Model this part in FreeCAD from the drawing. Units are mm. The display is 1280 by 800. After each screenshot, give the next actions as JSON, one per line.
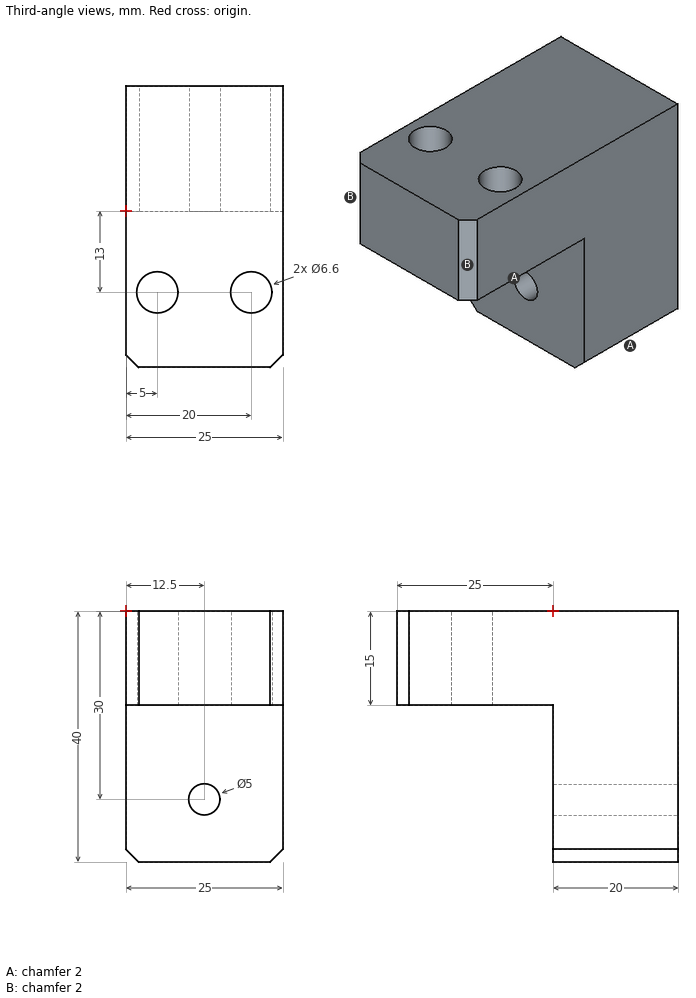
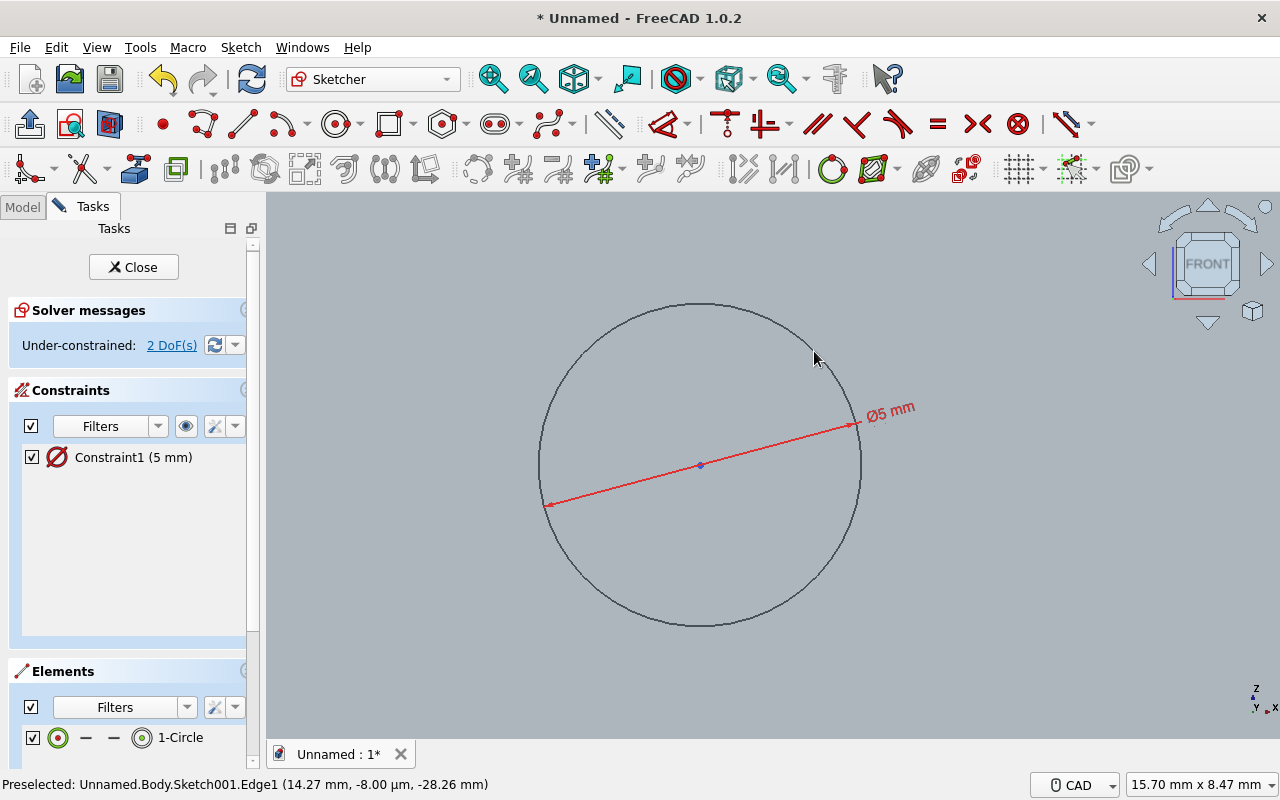
{"action": "left_click", "coordinate": [700, 465]}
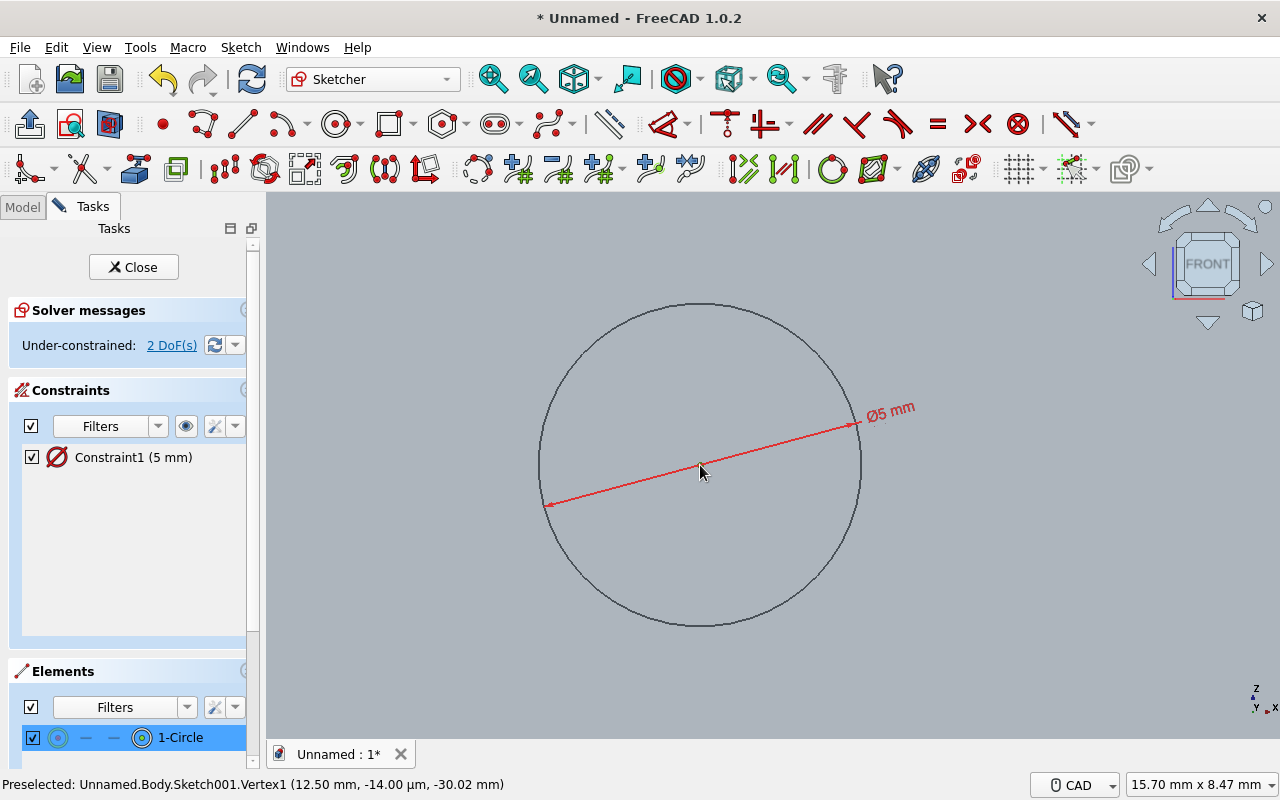
{"action": "key", "text": "i"}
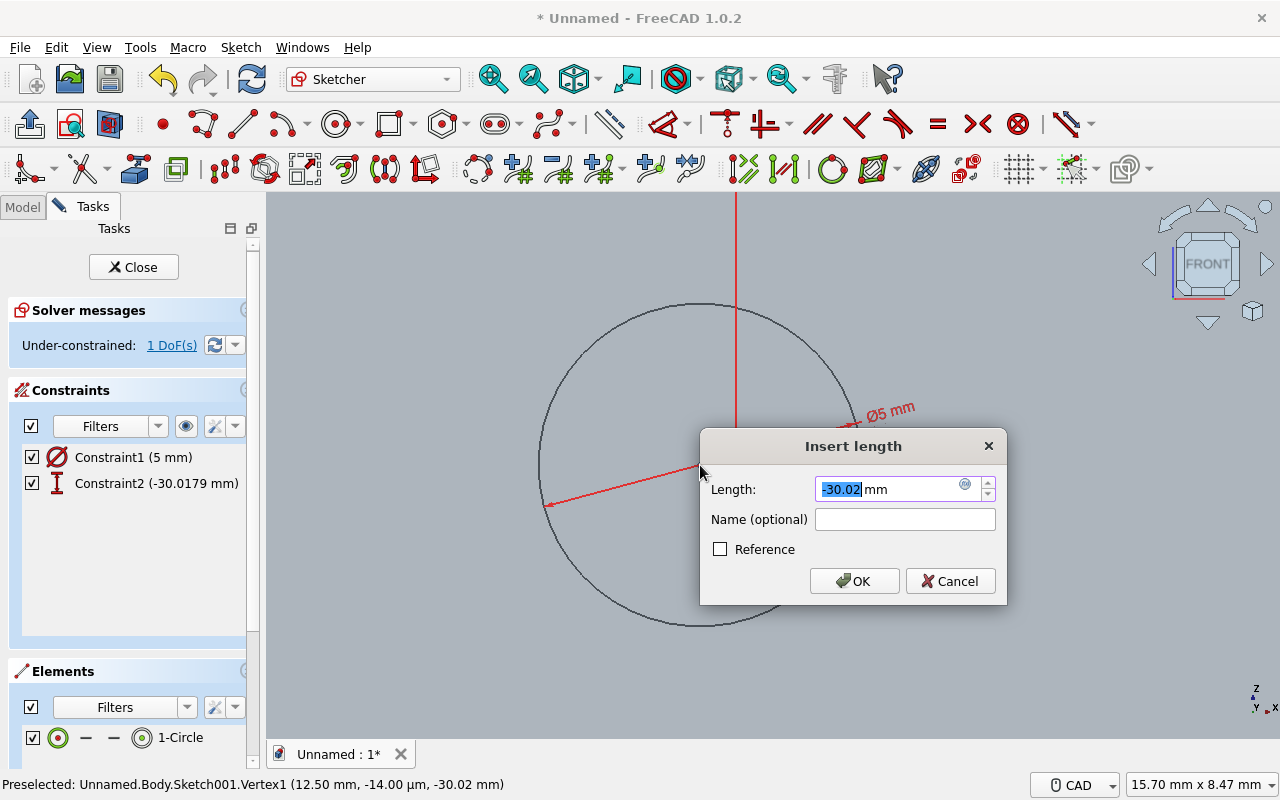
{"action": "type", "text": "-30"}
{"action": "key", "text": "Return"}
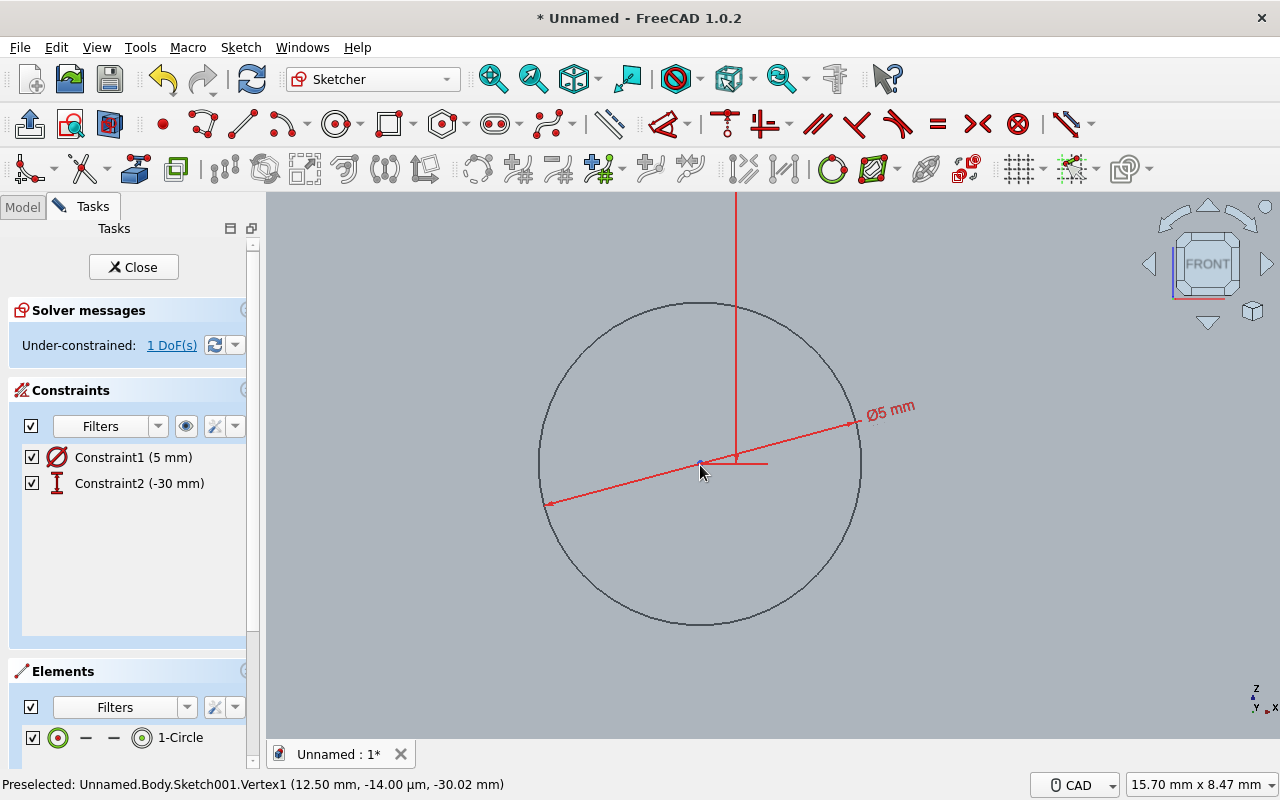
{"action": "left_click", "coordinate": [700, 464]}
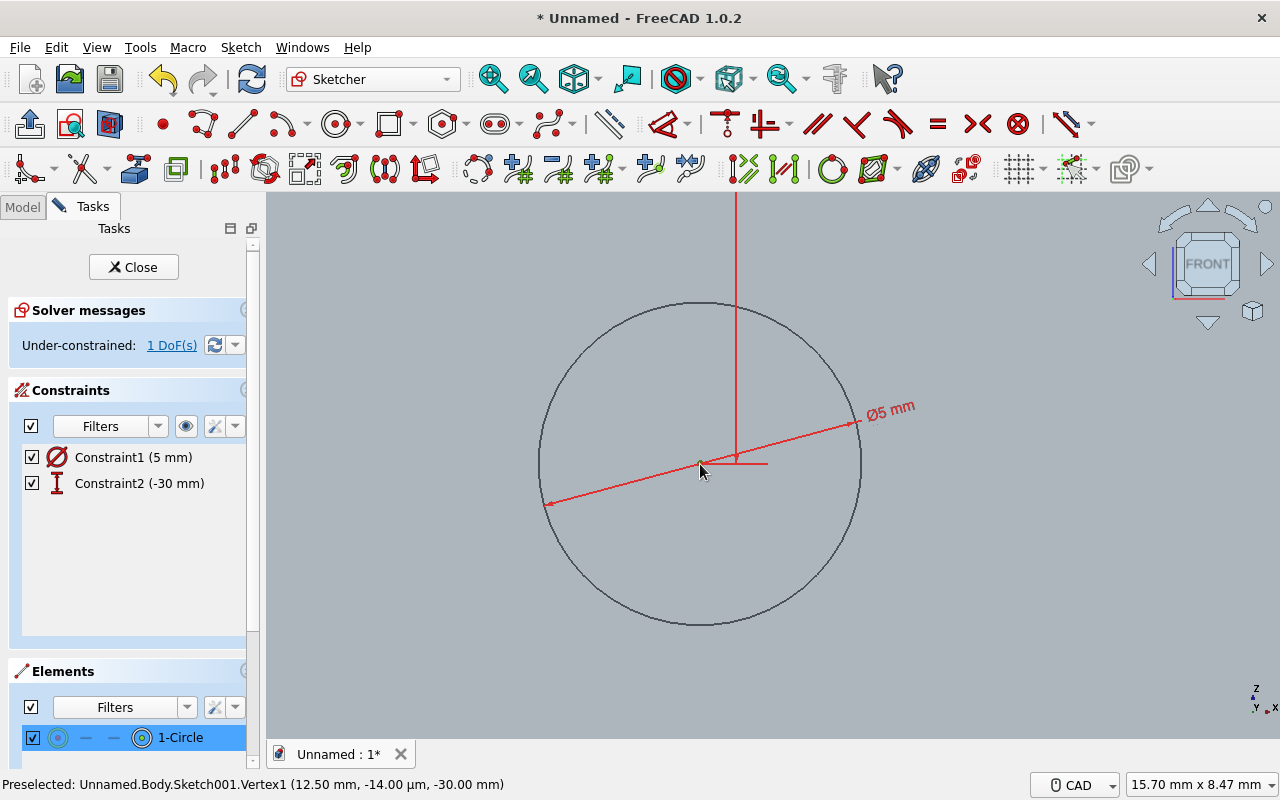
{"action": "key", "text": "l"}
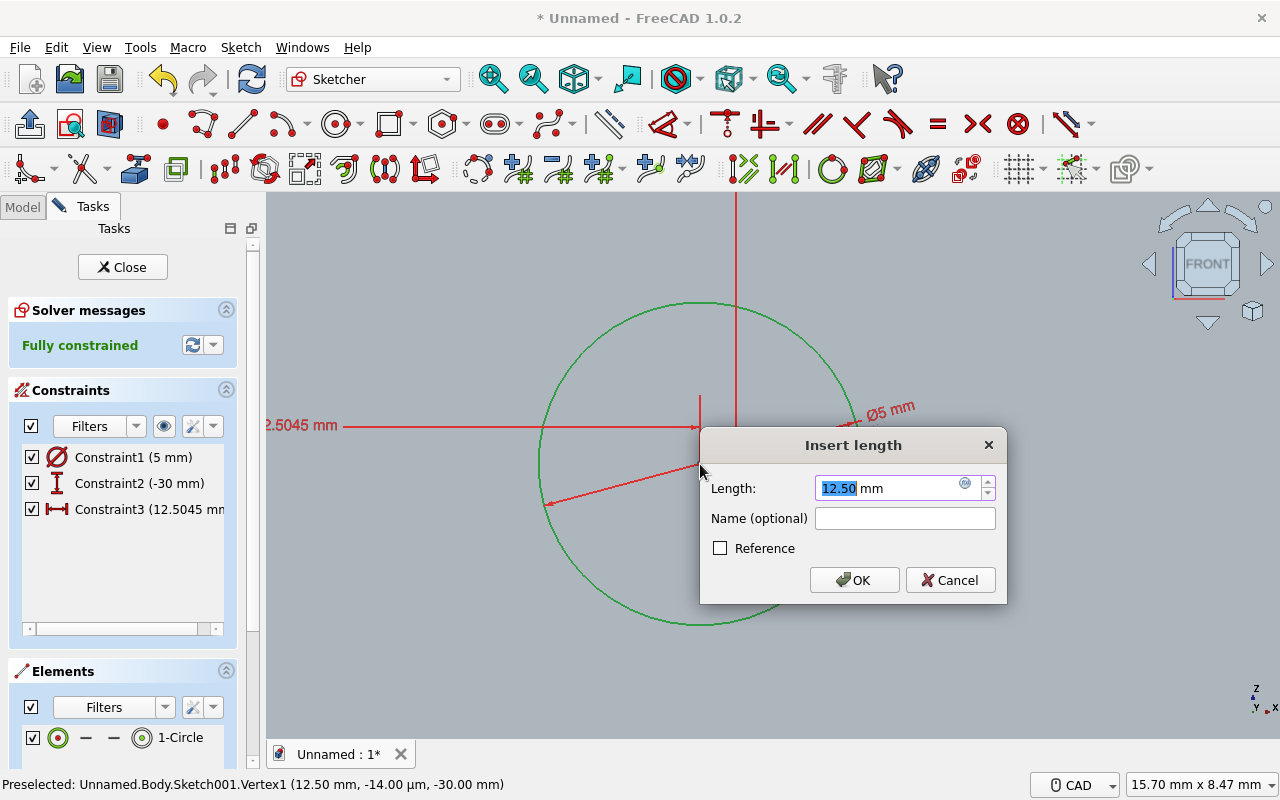
{"action": "type", "text": "12.5"}
{"action": "key", "text": "Return"}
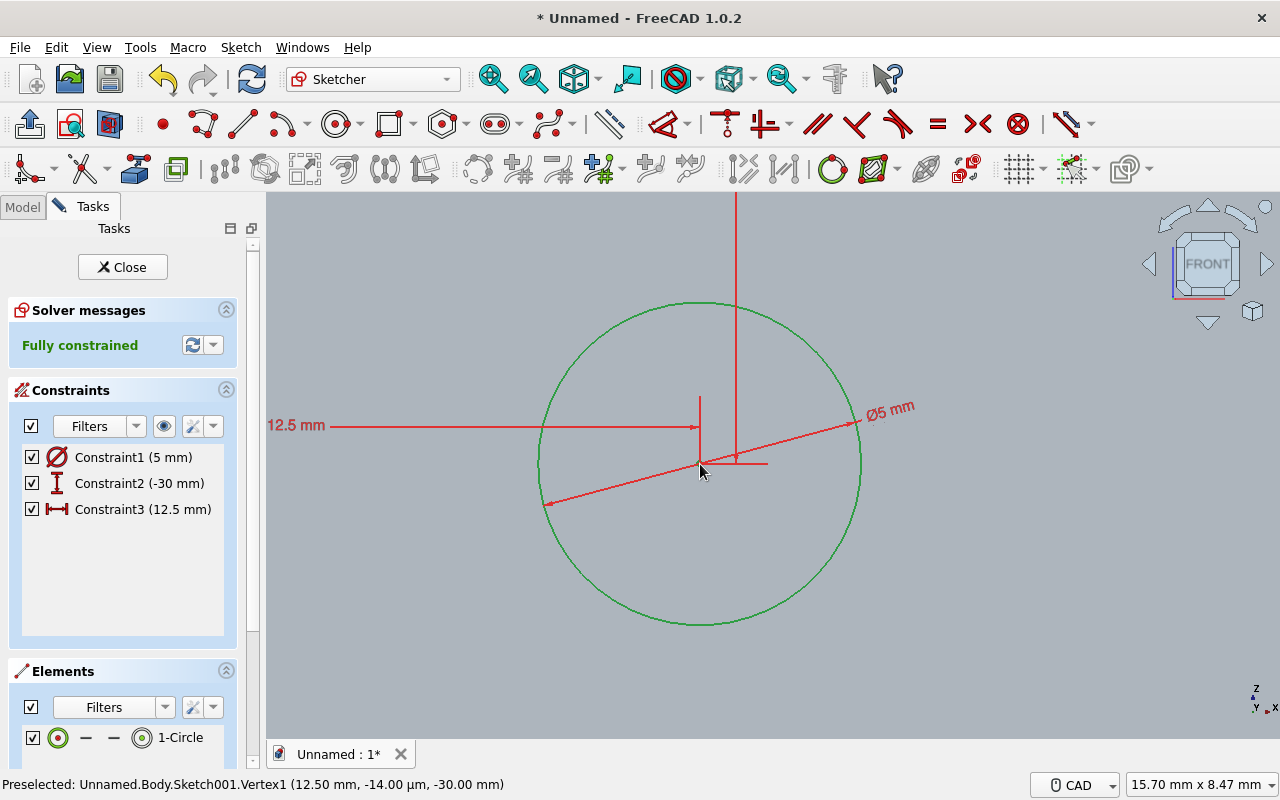
{"action": "left_click", "coordinate": [123, 267]}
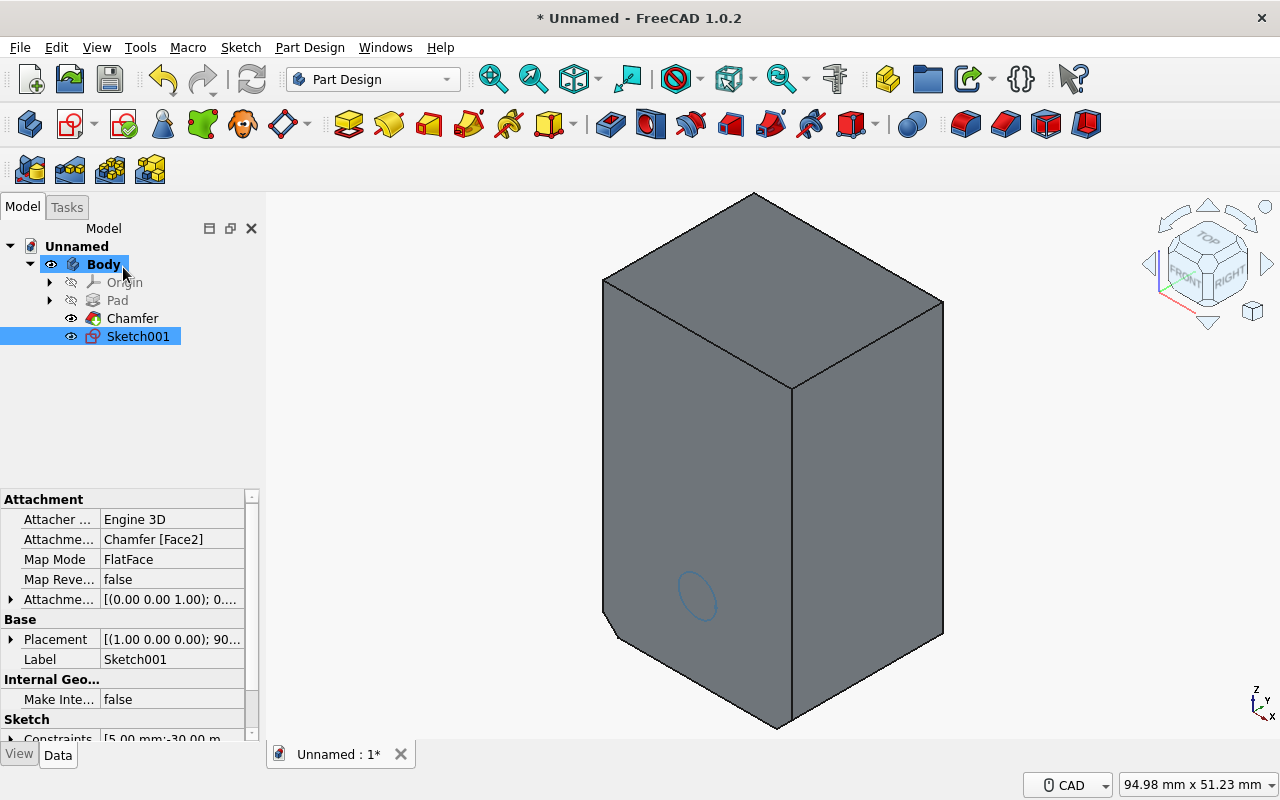
{"action": "left_click", "coordinate": [612, 124]}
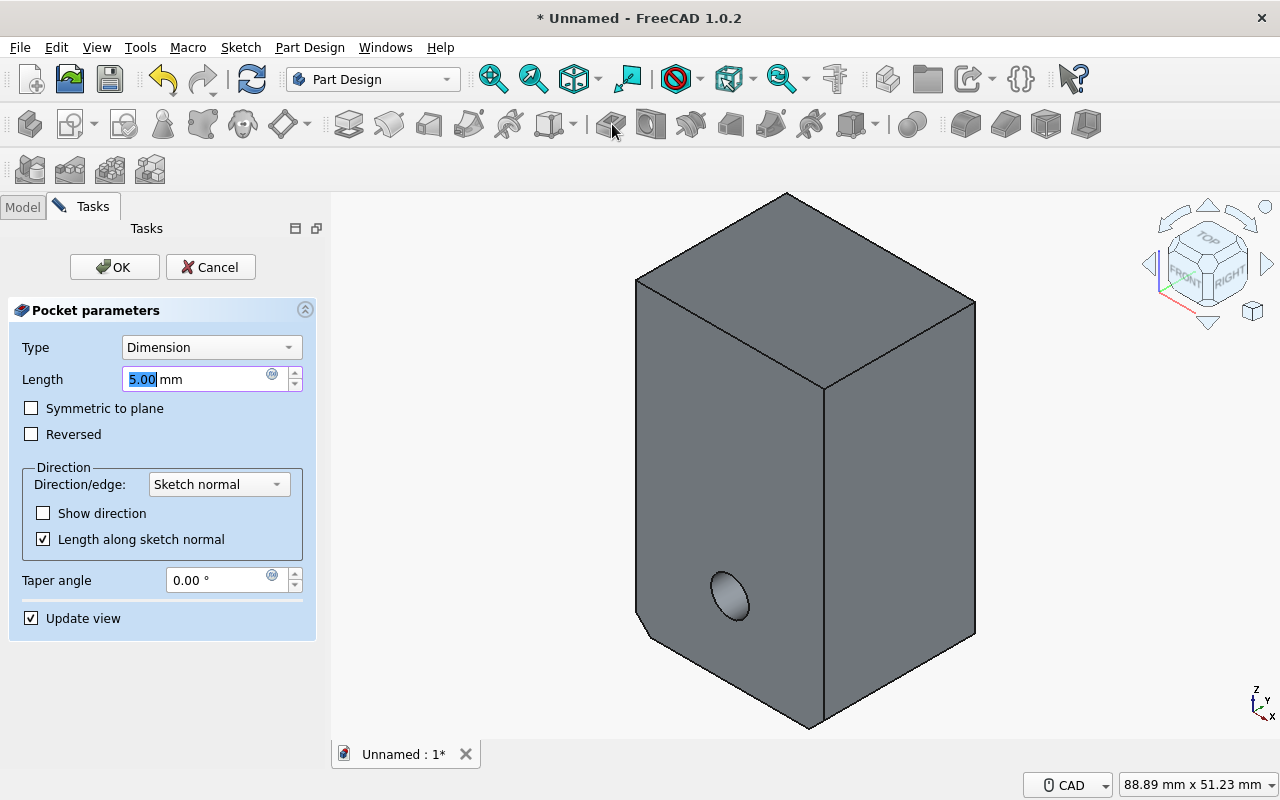
{"action": "left_click", "coordinate": [212, 348]}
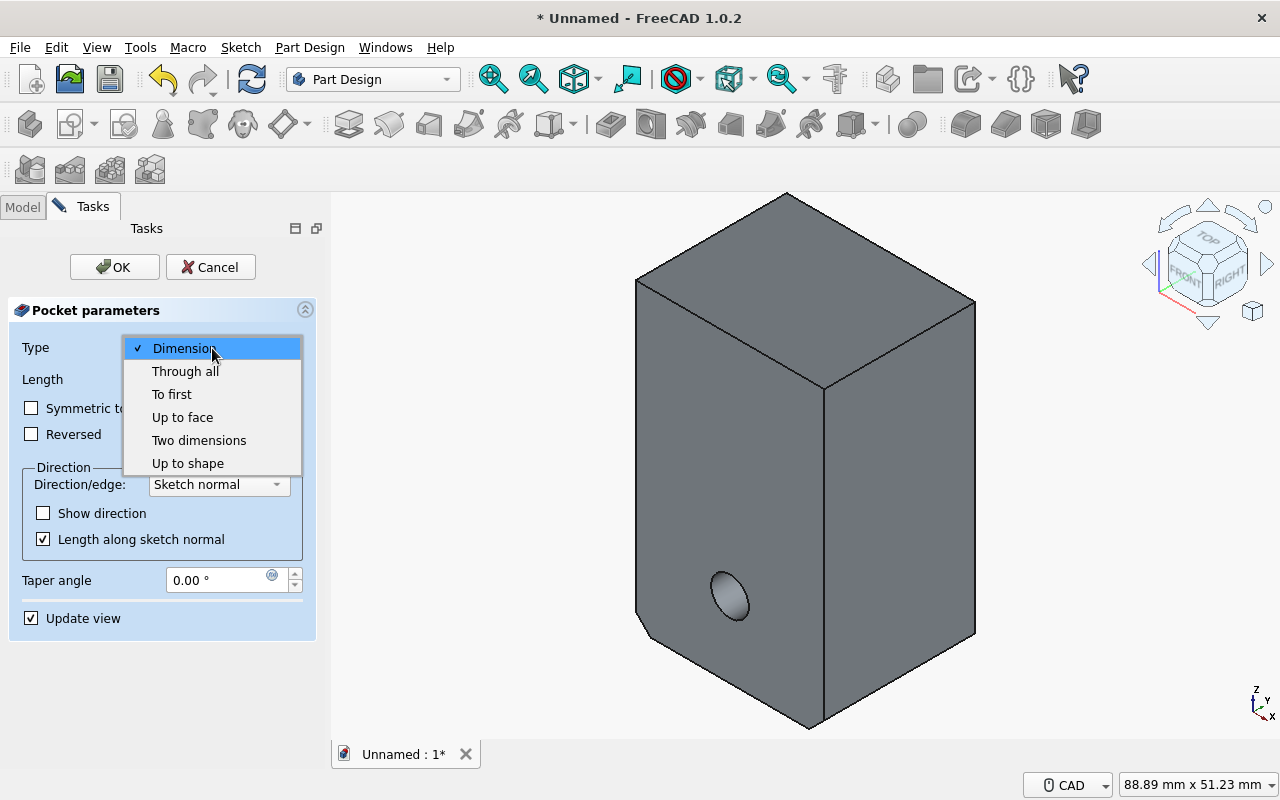
{"action": "left_click", "coordinate": [212, 372]}